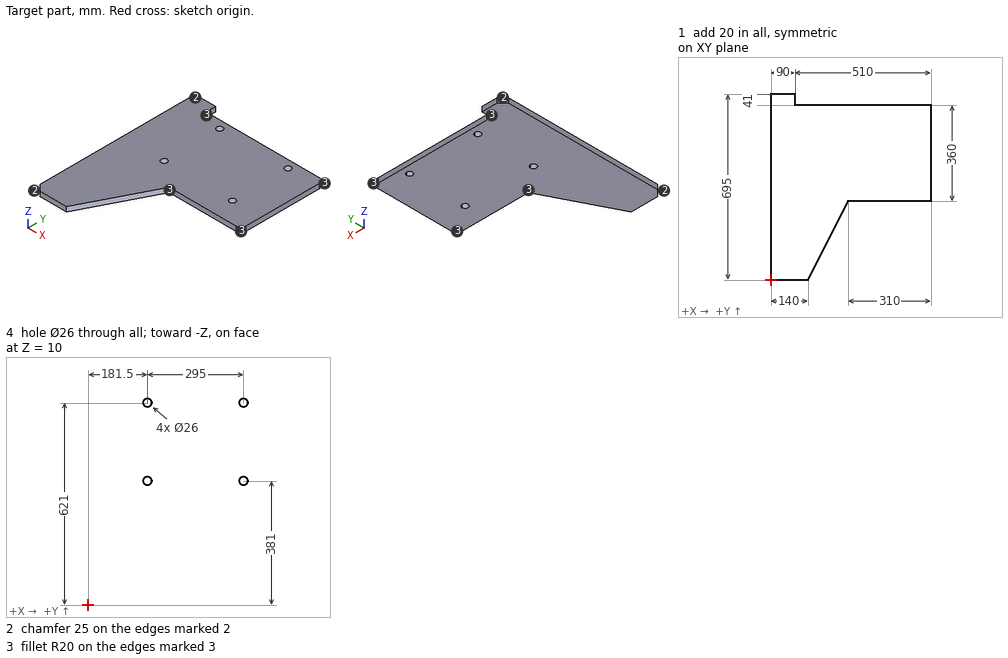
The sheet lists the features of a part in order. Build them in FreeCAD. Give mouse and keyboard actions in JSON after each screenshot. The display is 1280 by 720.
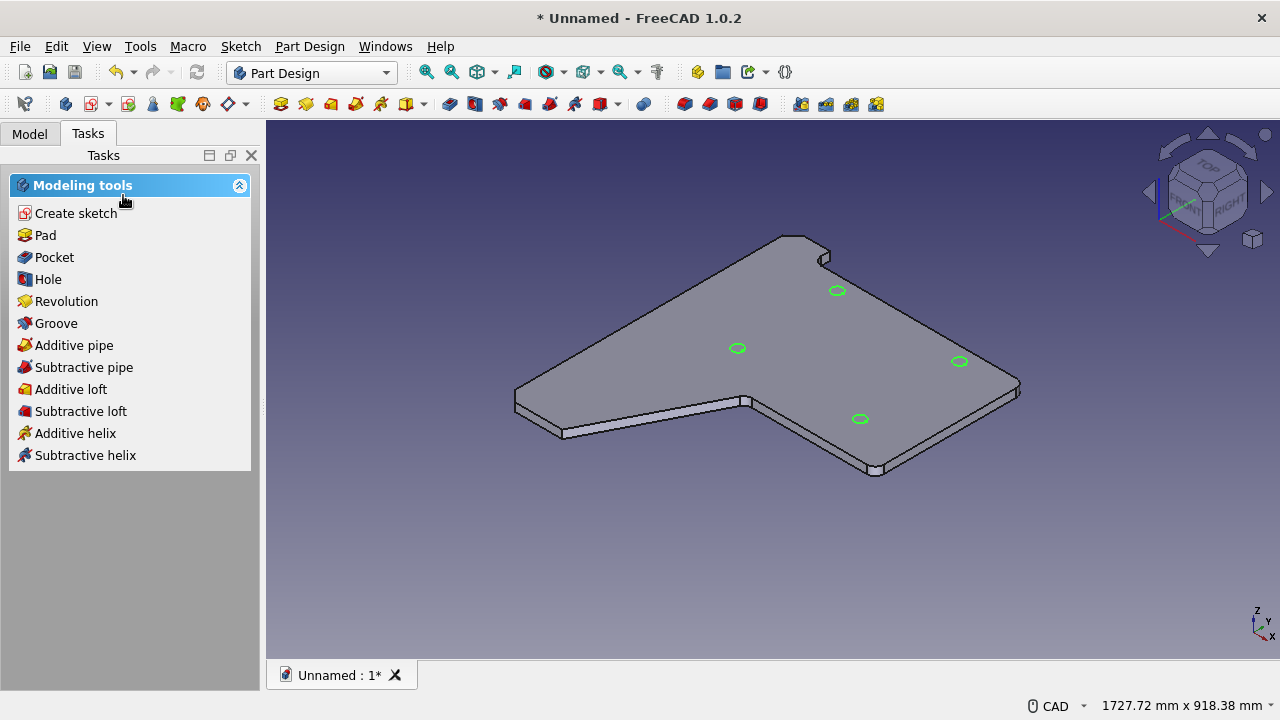
{"action": "left_click", "coordinate": [475, 104]}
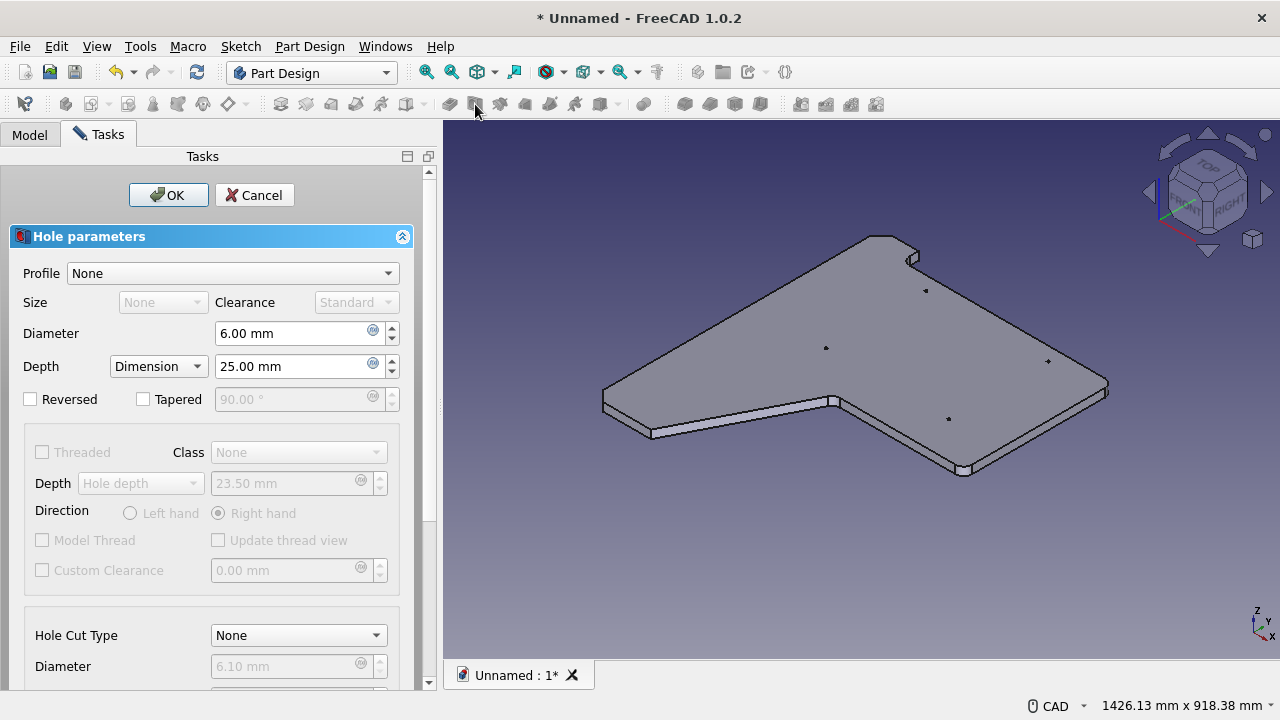
{"action": "triple_click", "coordinate": [300, 334]}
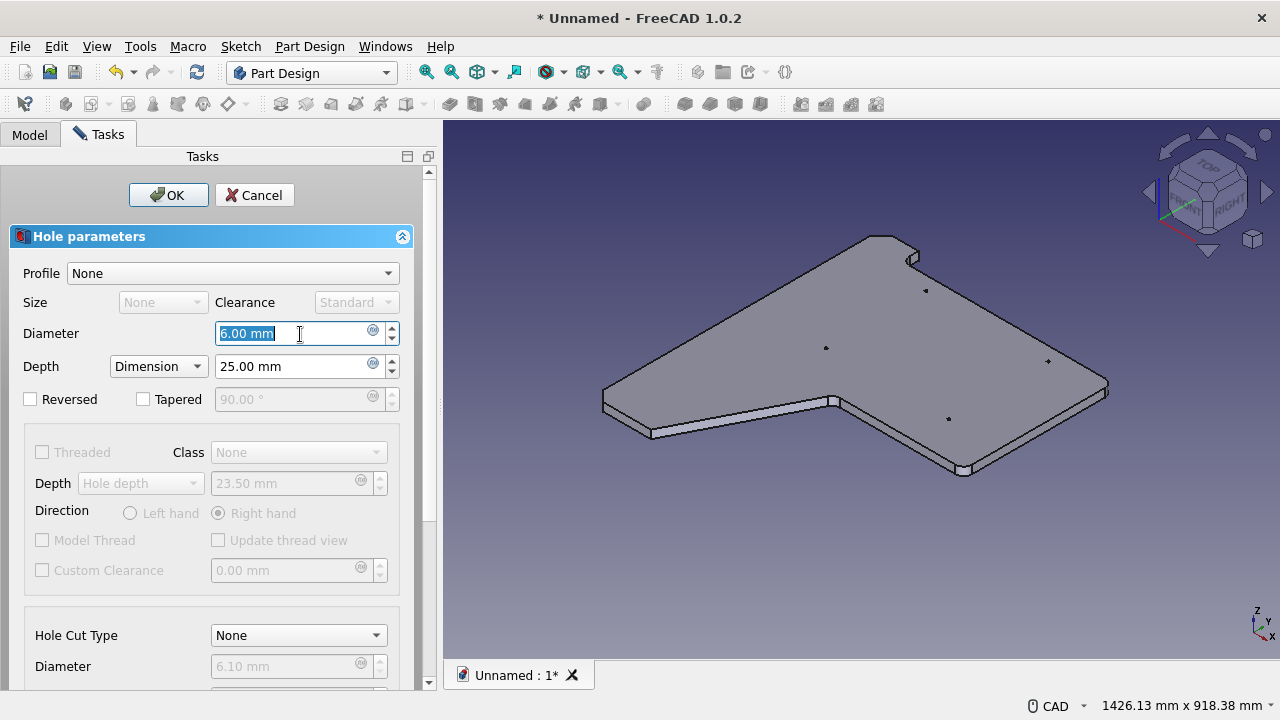
{"action": "type", "text": "26"}
{"action": "key", "text": "Tab"}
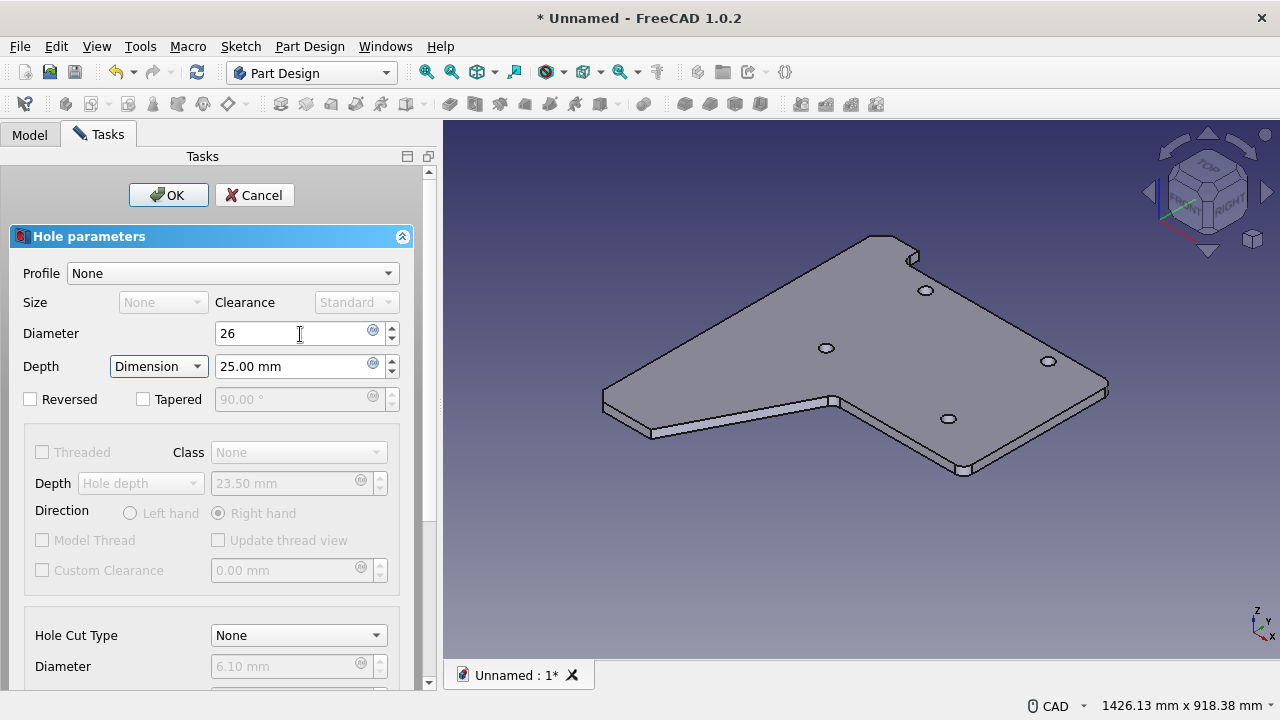
{"action": "left_click", "coordinate": [160, 366]}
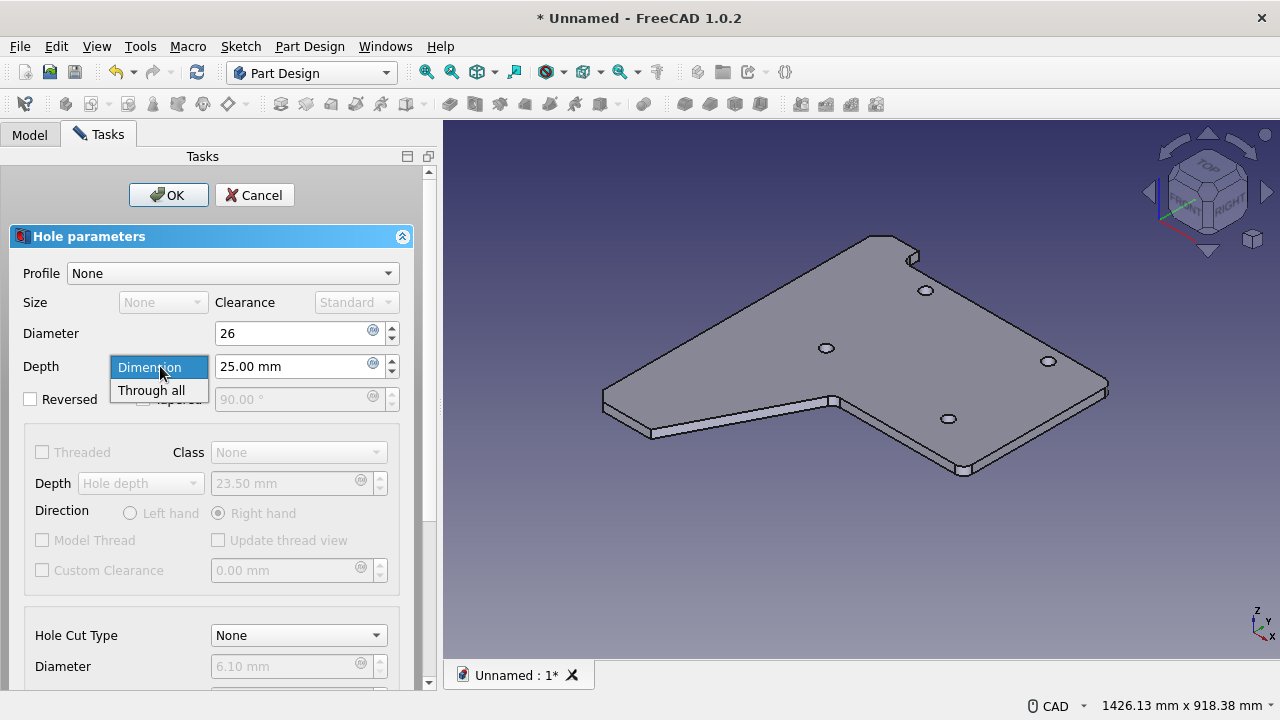
{"action": "left_click", "coordinate": [158, 390]}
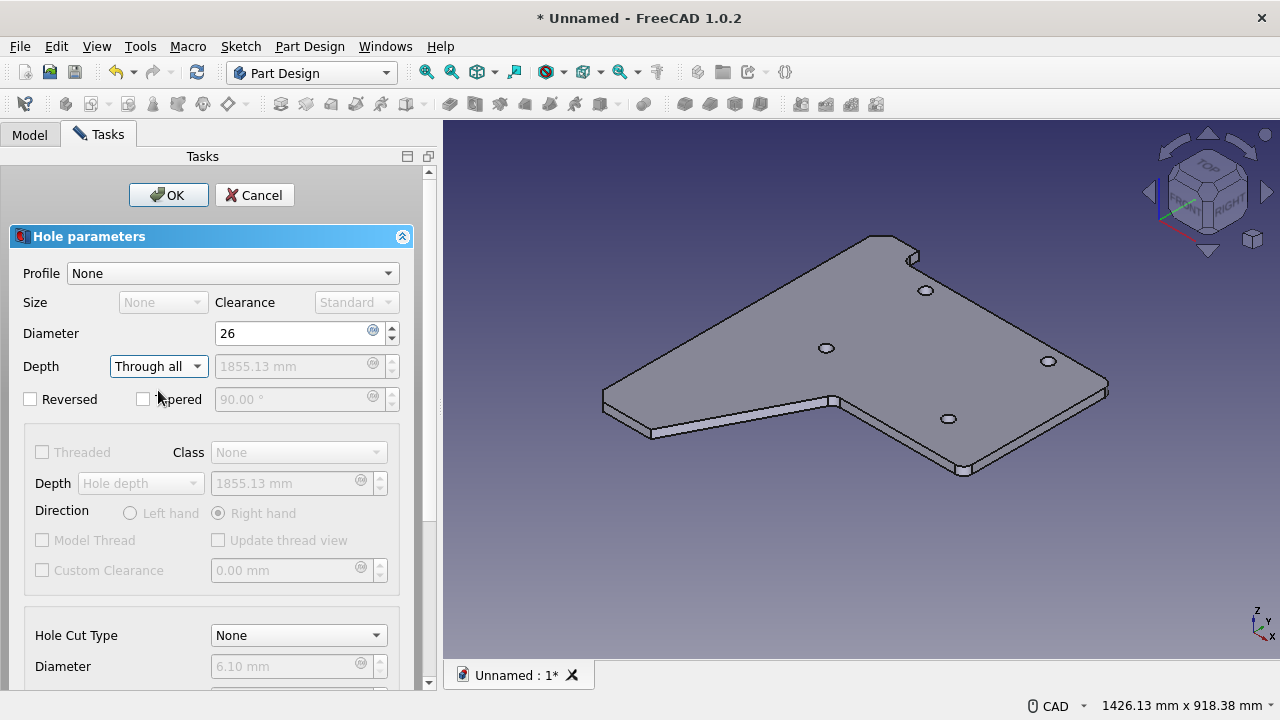
{"action": "left_click", "coordinate": [169, 195]}